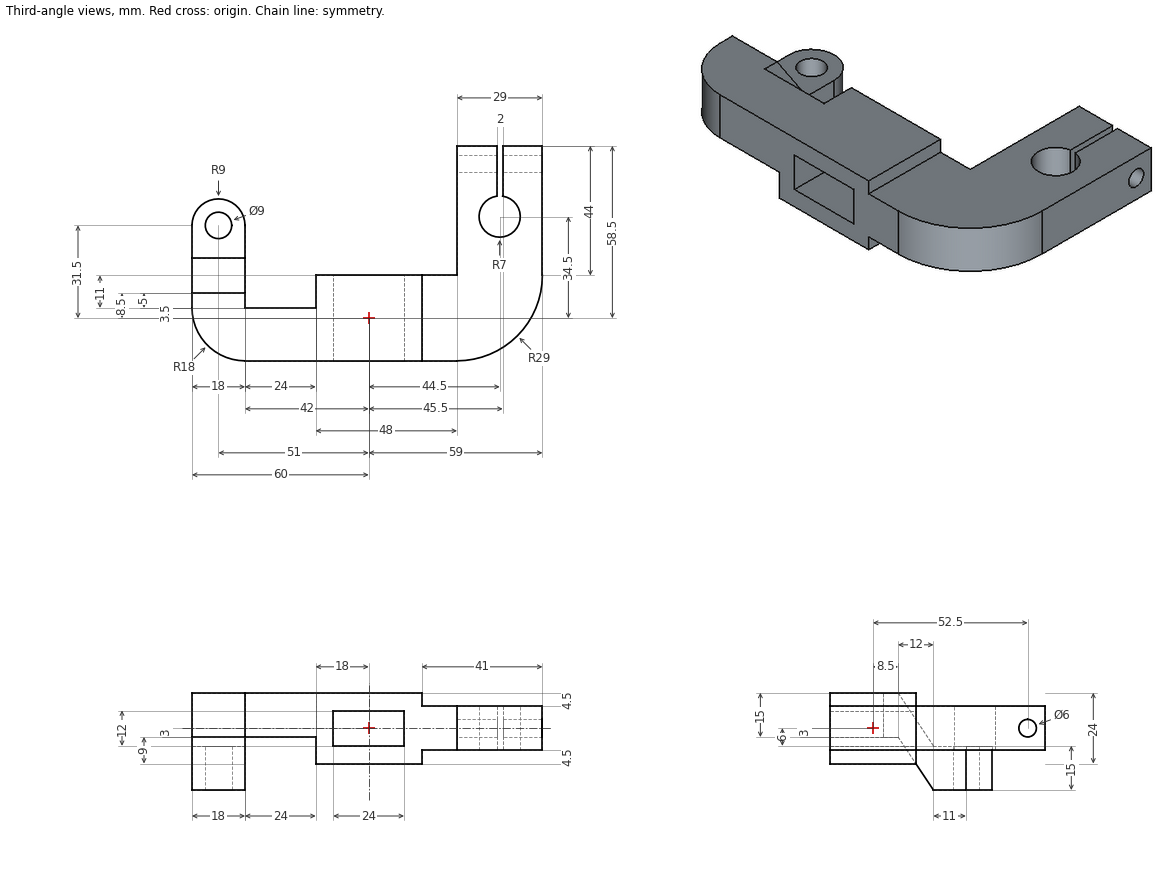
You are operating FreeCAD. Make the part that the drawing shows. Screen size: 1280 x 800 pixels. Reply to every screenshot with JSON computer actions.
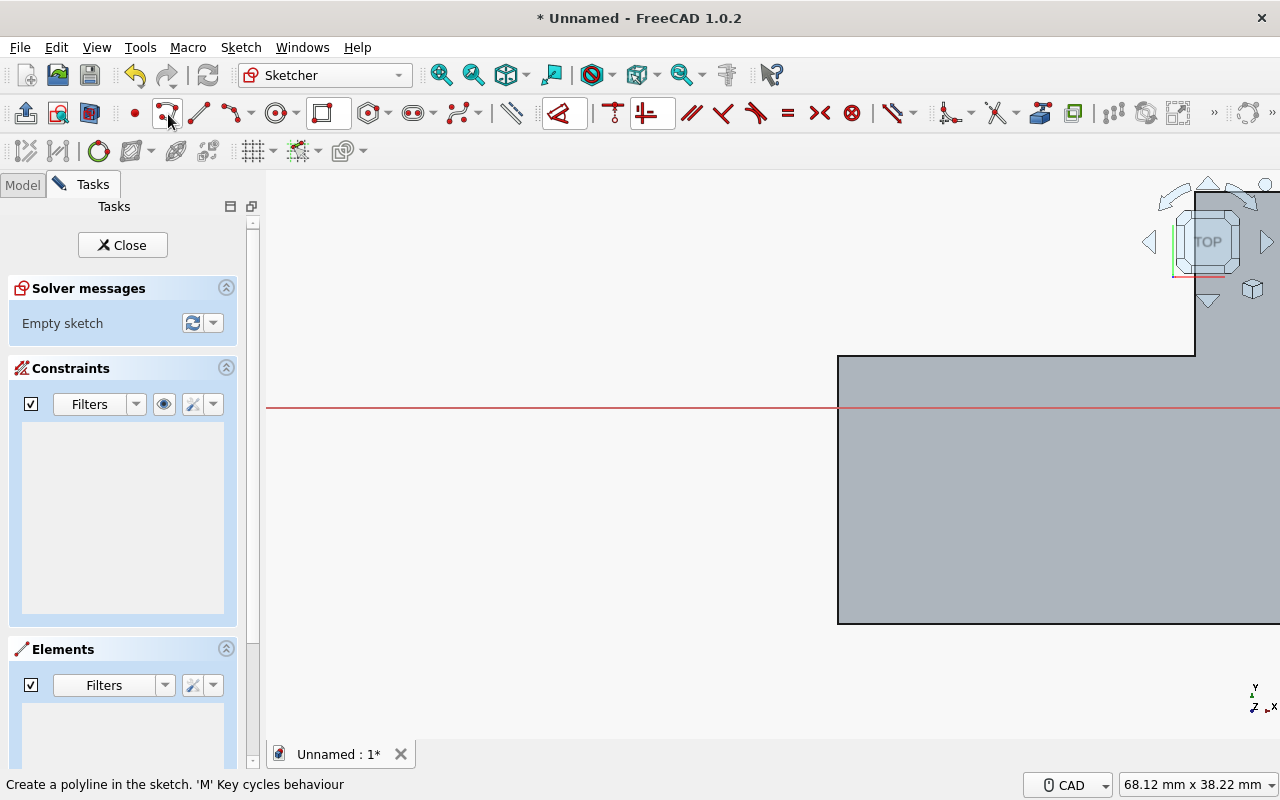
{"action": "left_click", "coordinate": [838, 624]}
{"action": "left_click", "coordinate": [838, 281]}
{"action": "left_click", "coordinate": [570, 281]}
{"action": "left_click", "coordinate": [570, 356]}
{"action": "right_click", "coordinate": [570, 356]}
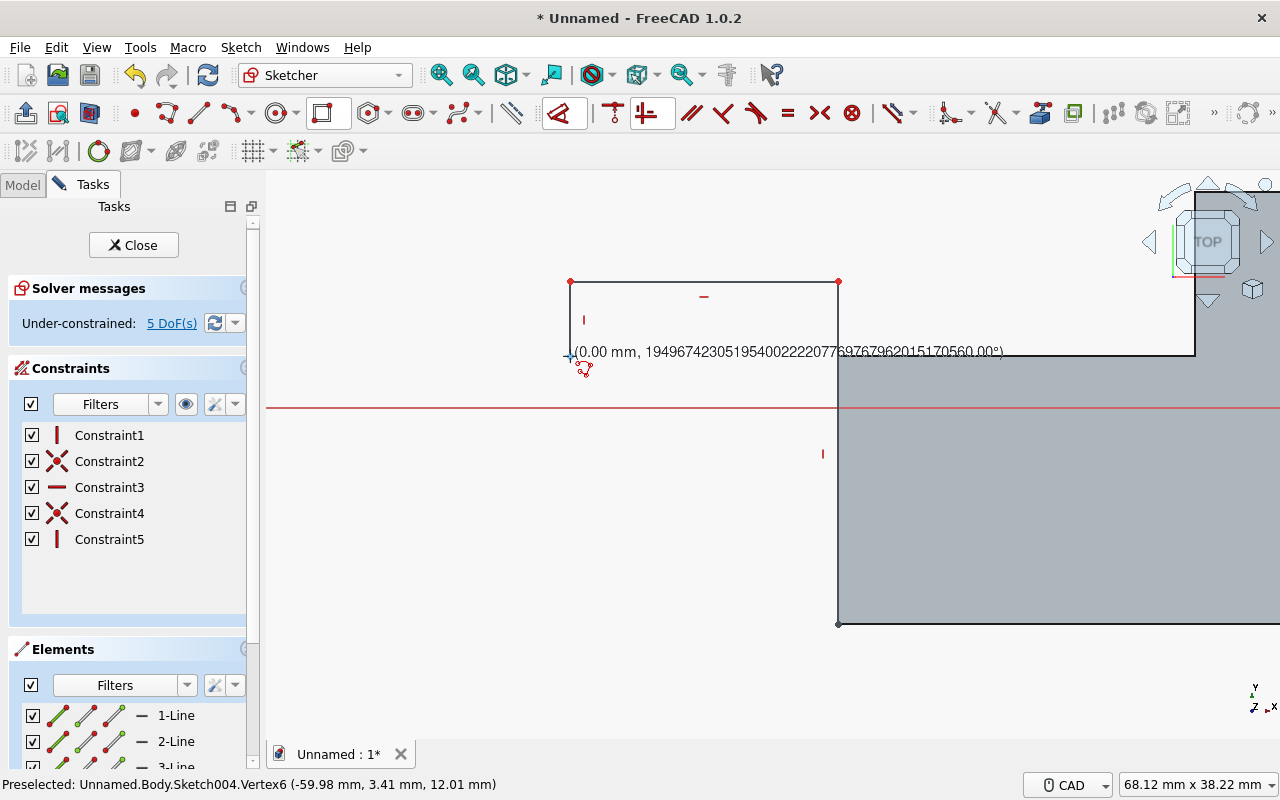
{"action": "left_click", "coordinate": [232, 114]}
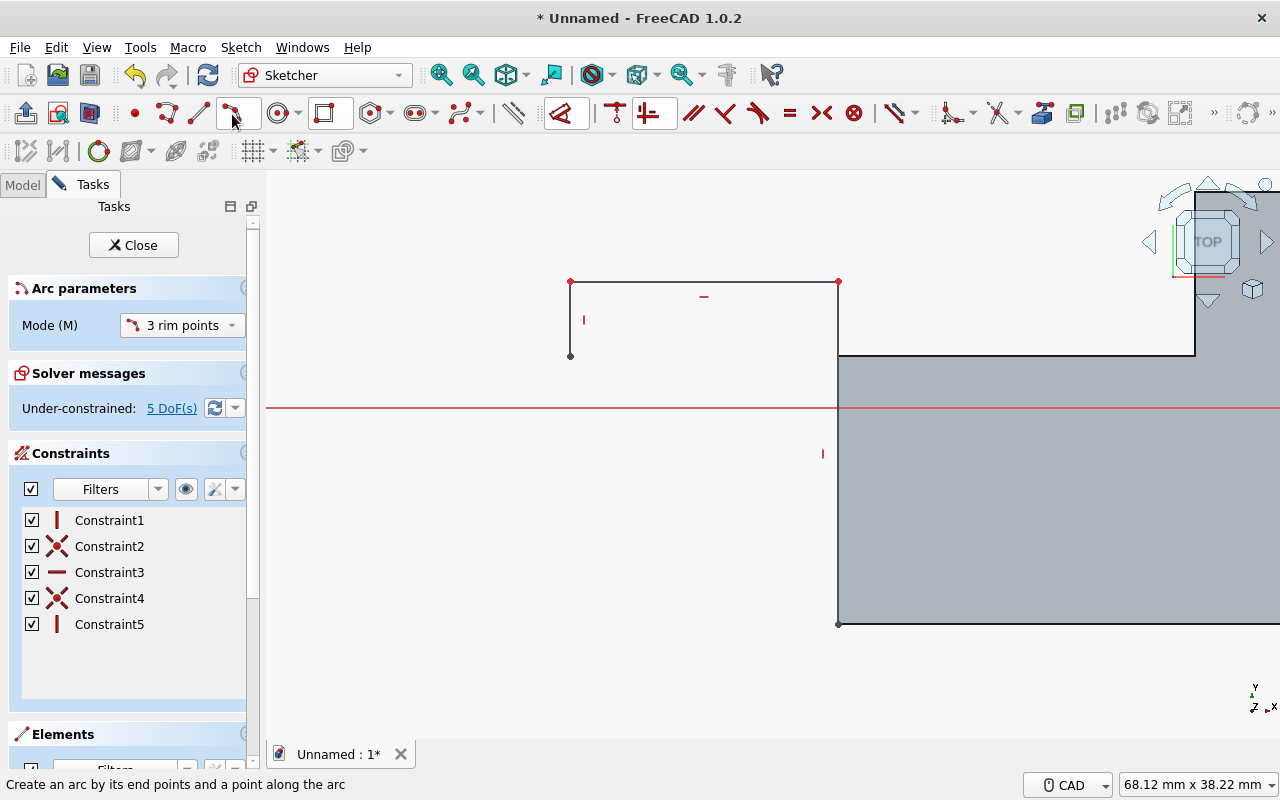
{"action": "left_click", "coordinate": [570, 357]}
{"action": "left_click", "coordinate": [838, 625]}
{"action": "left_click", "coordinate": [648, 545]}
{"action": "key", "text": "Escape"}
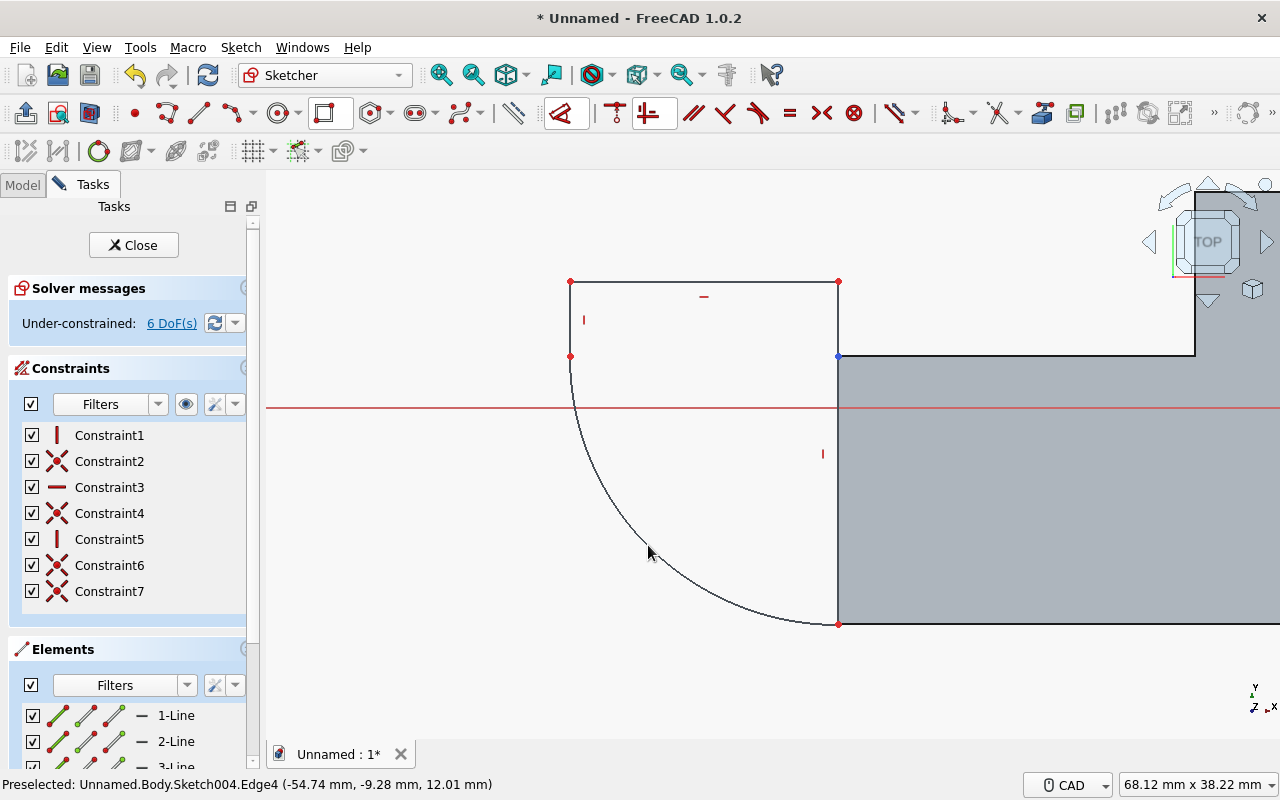
{"action": "left_click", "coordinate": [570, 304]}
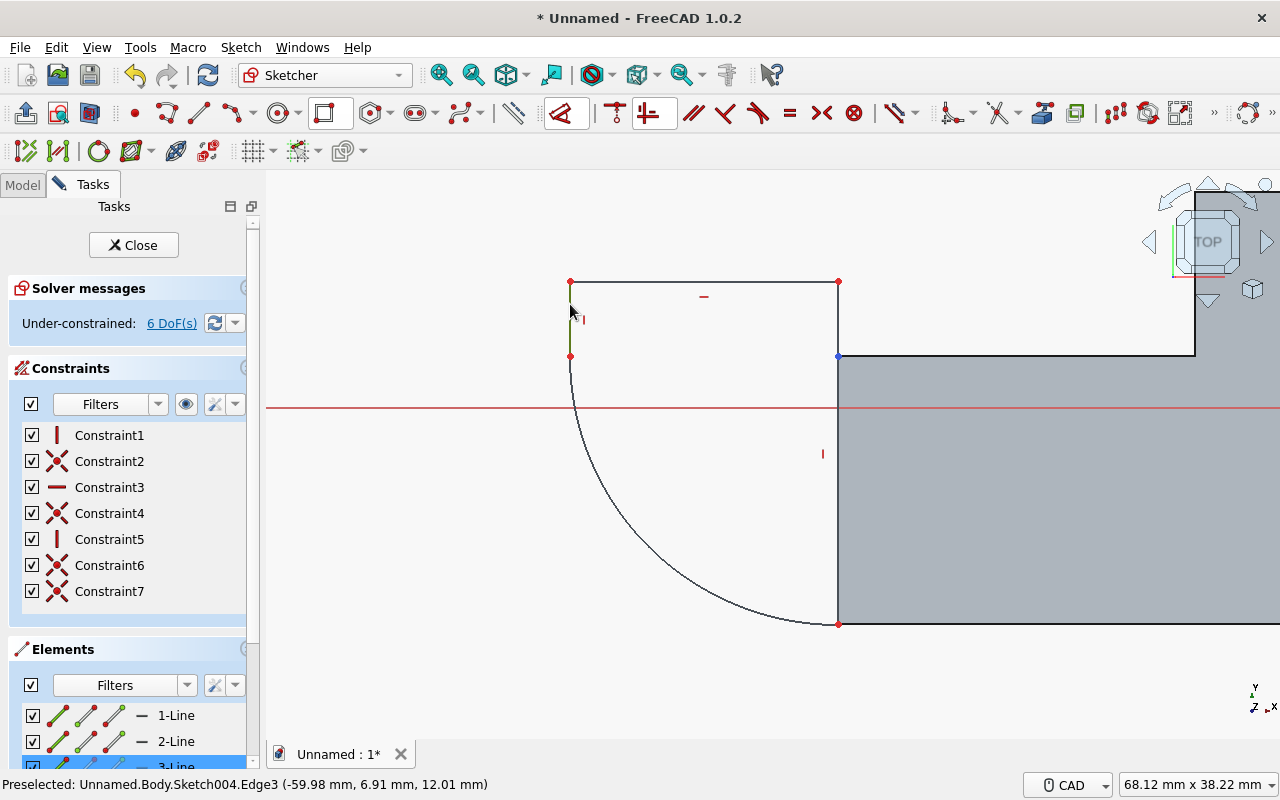
{"action": "left_click", "coordinate": [599, 479]}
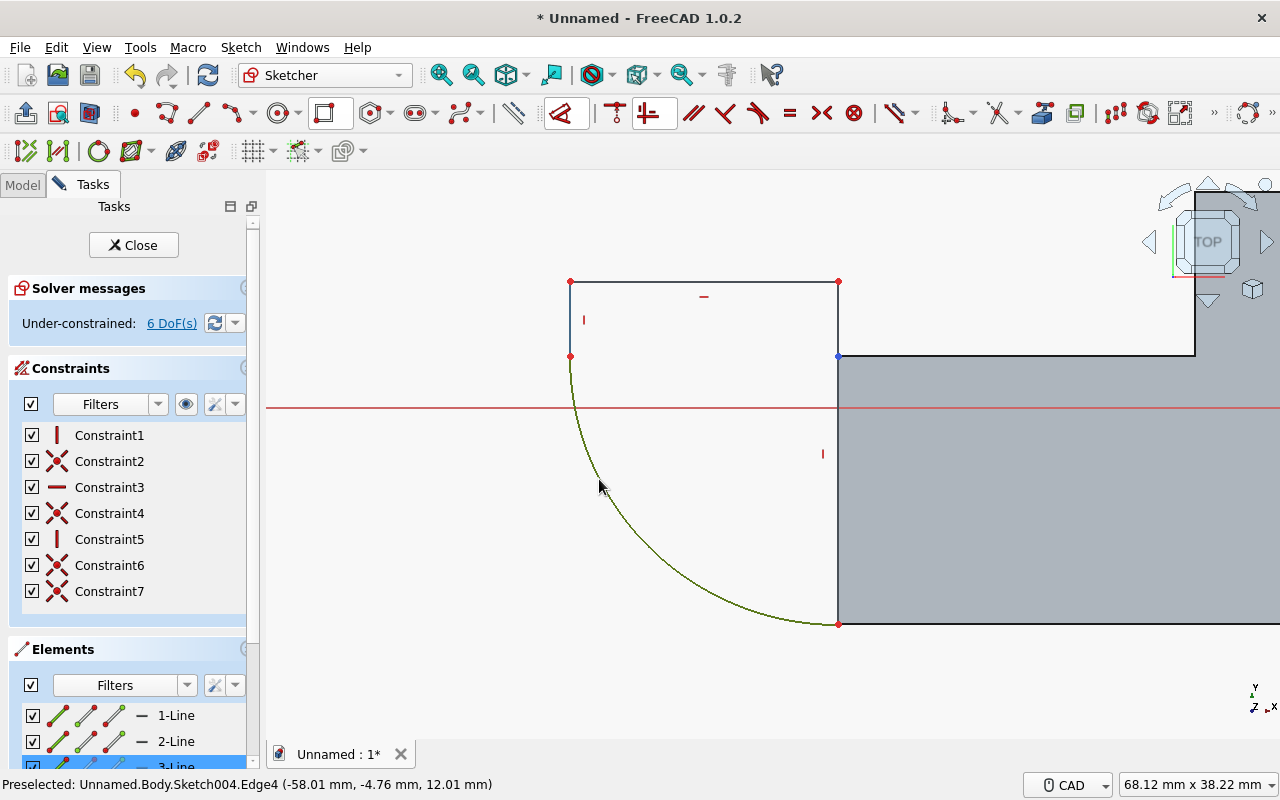
{"action": "left_click", "coordinate": [758, 114]}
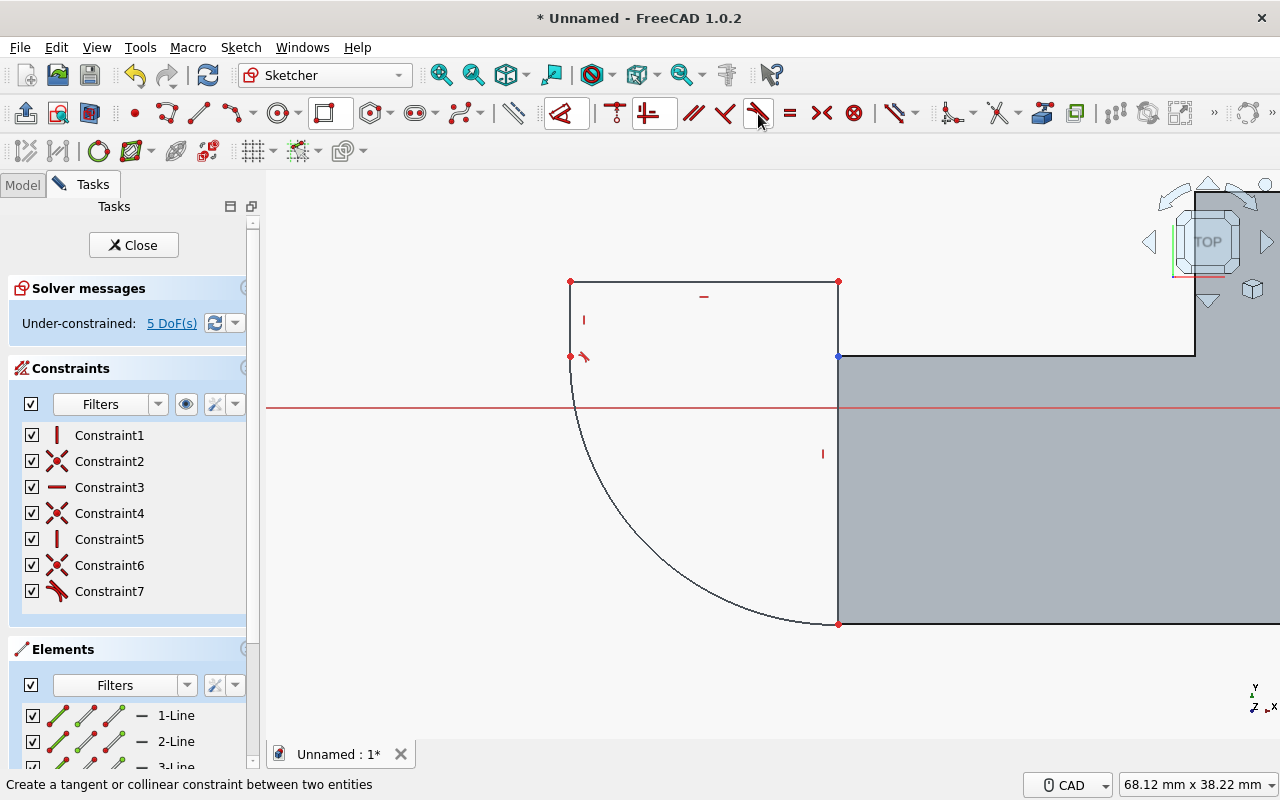
{"action": "left_click", "coordinate": [599, 479]}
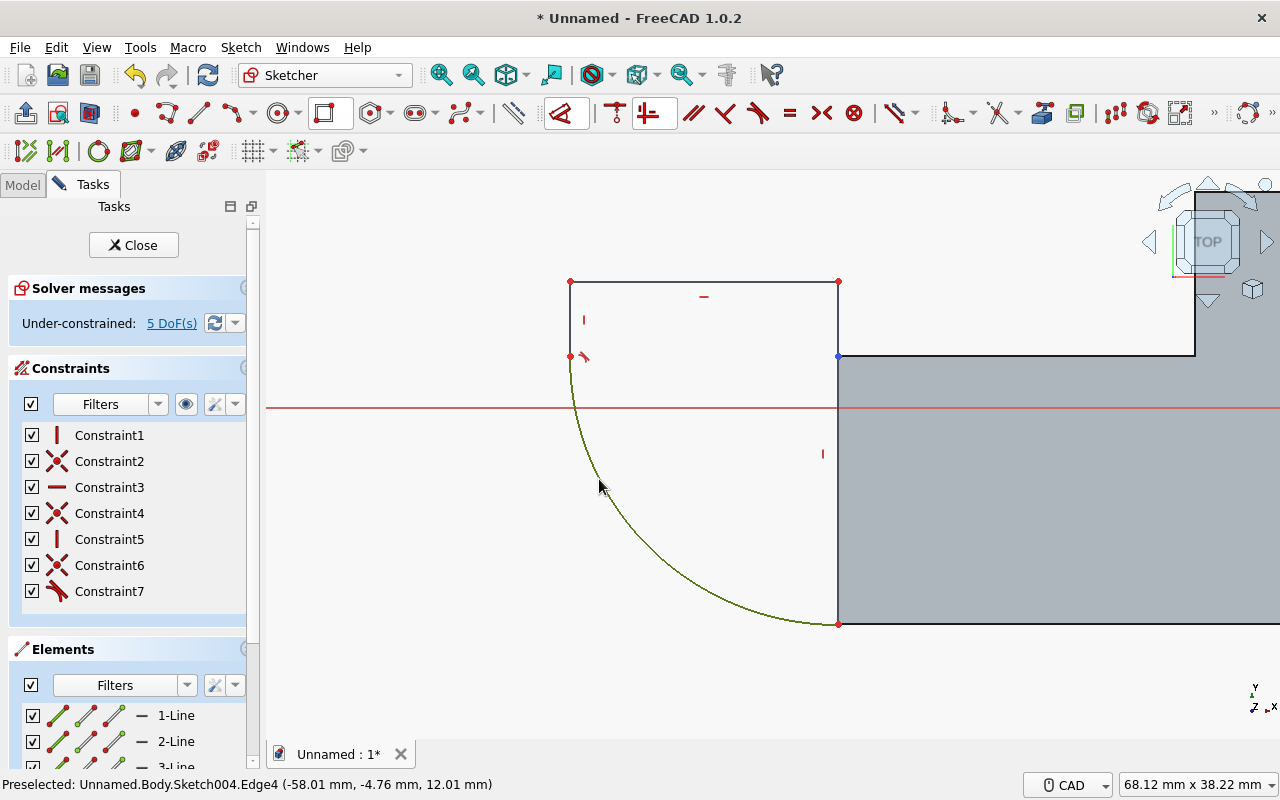
{"action": "key", "text": "k r"}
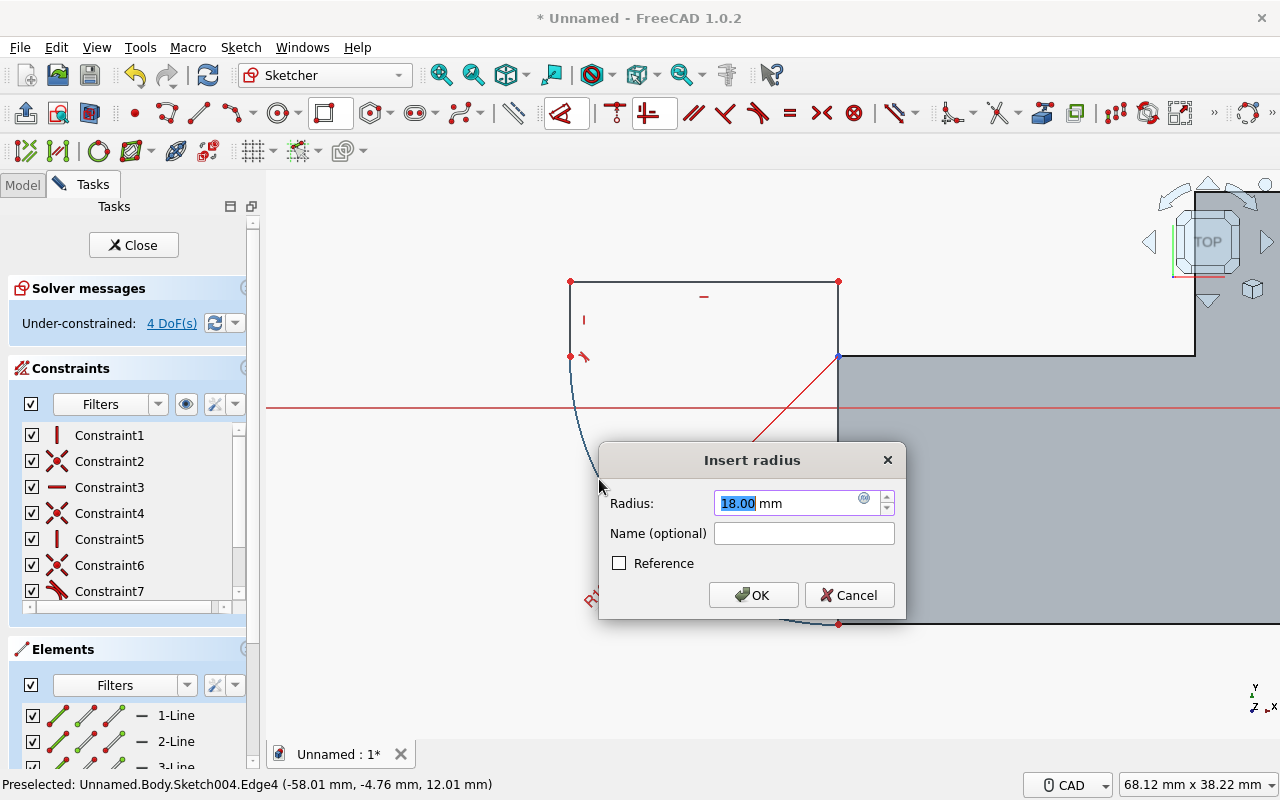
{"action": "type", "text": "18"}
{"action": "key", "text": "Return"}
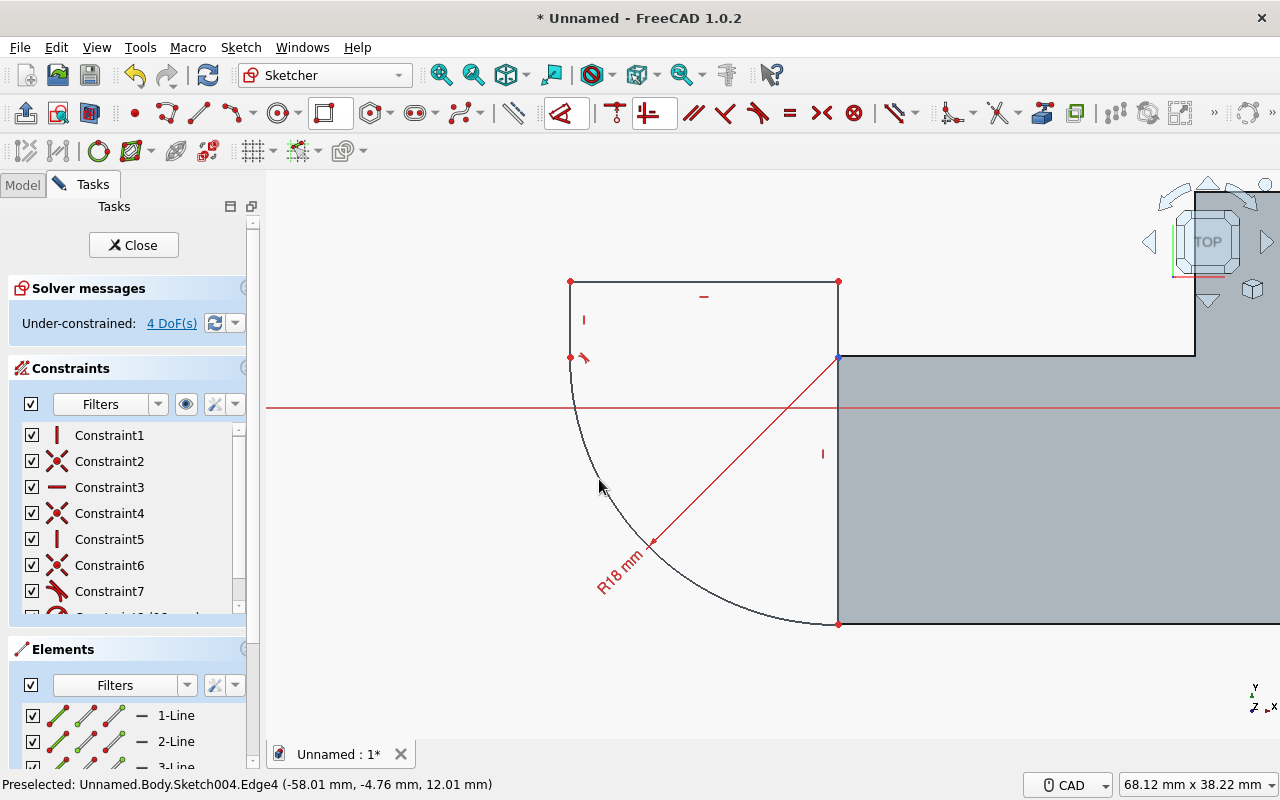
{"action": "left_click", "coordinate": [570, 305]}